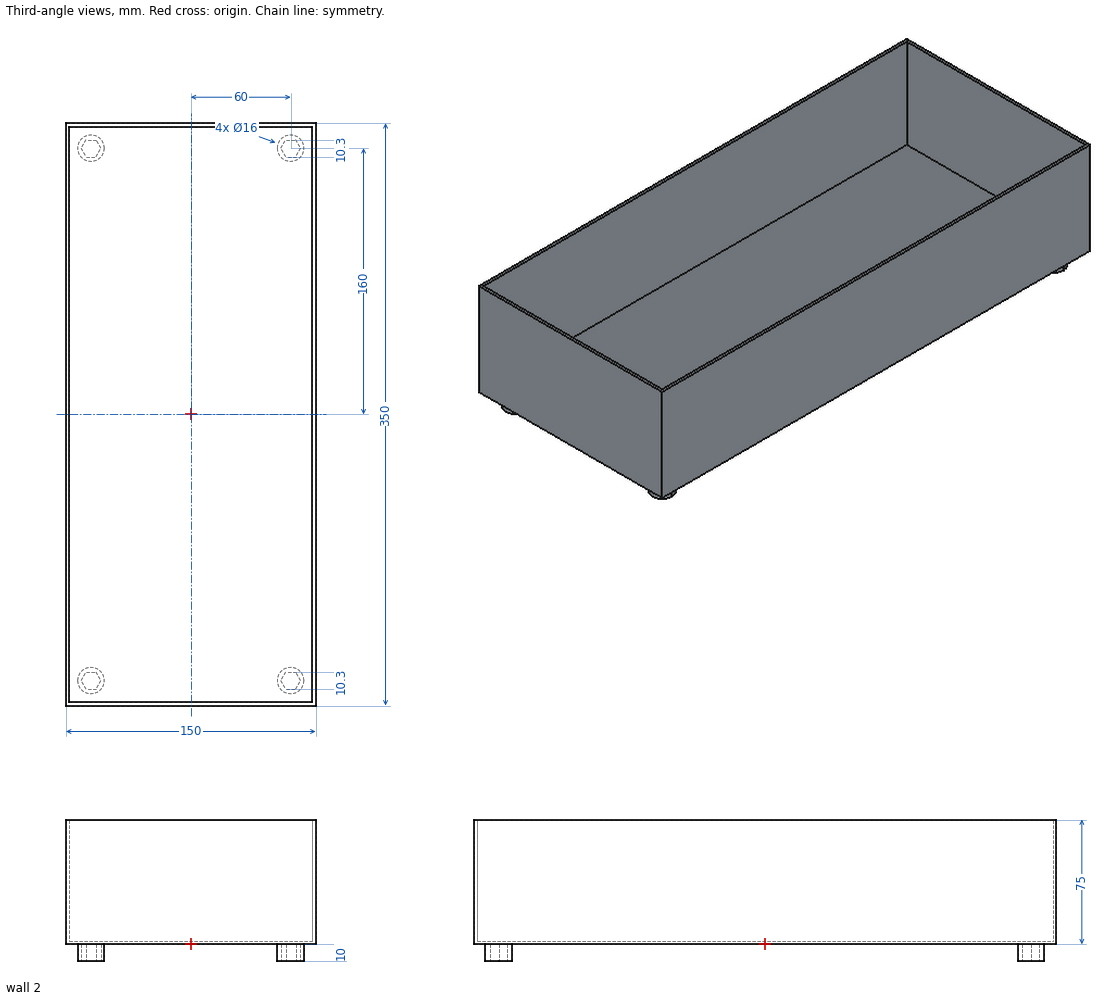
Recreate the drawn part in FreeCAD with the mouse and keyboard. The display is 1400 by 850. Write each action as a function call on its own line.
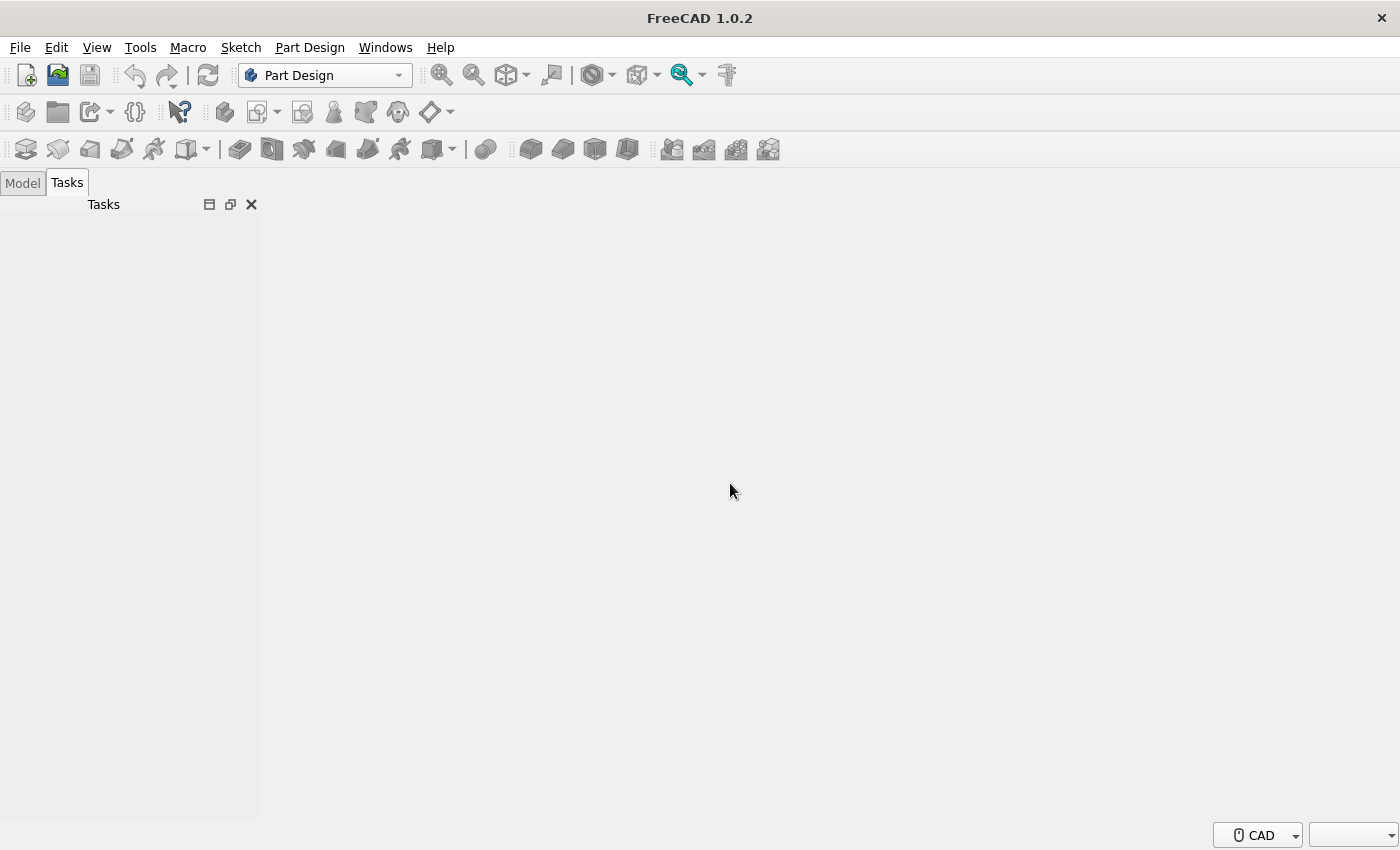
click(26, 76)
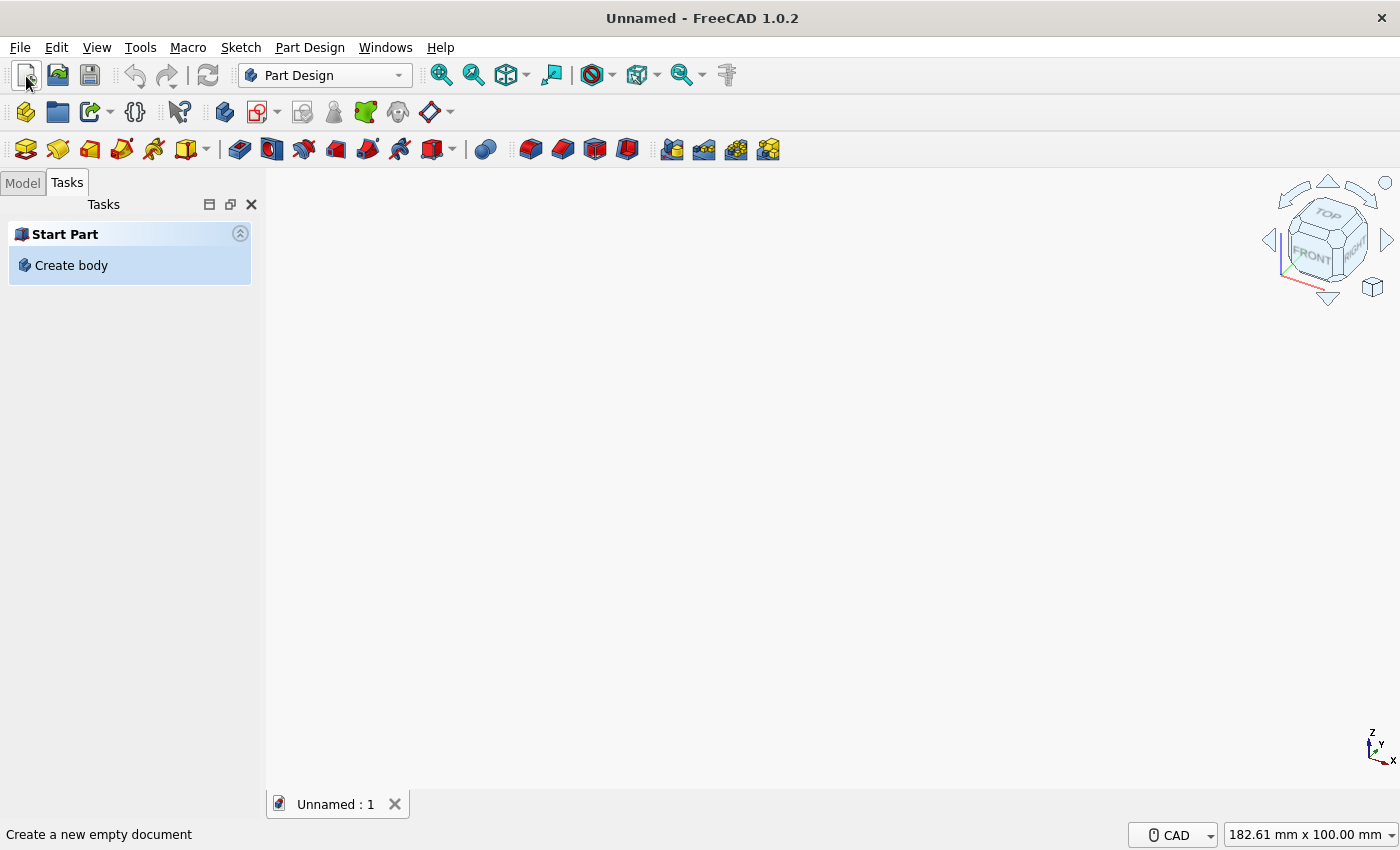
click(258, 112)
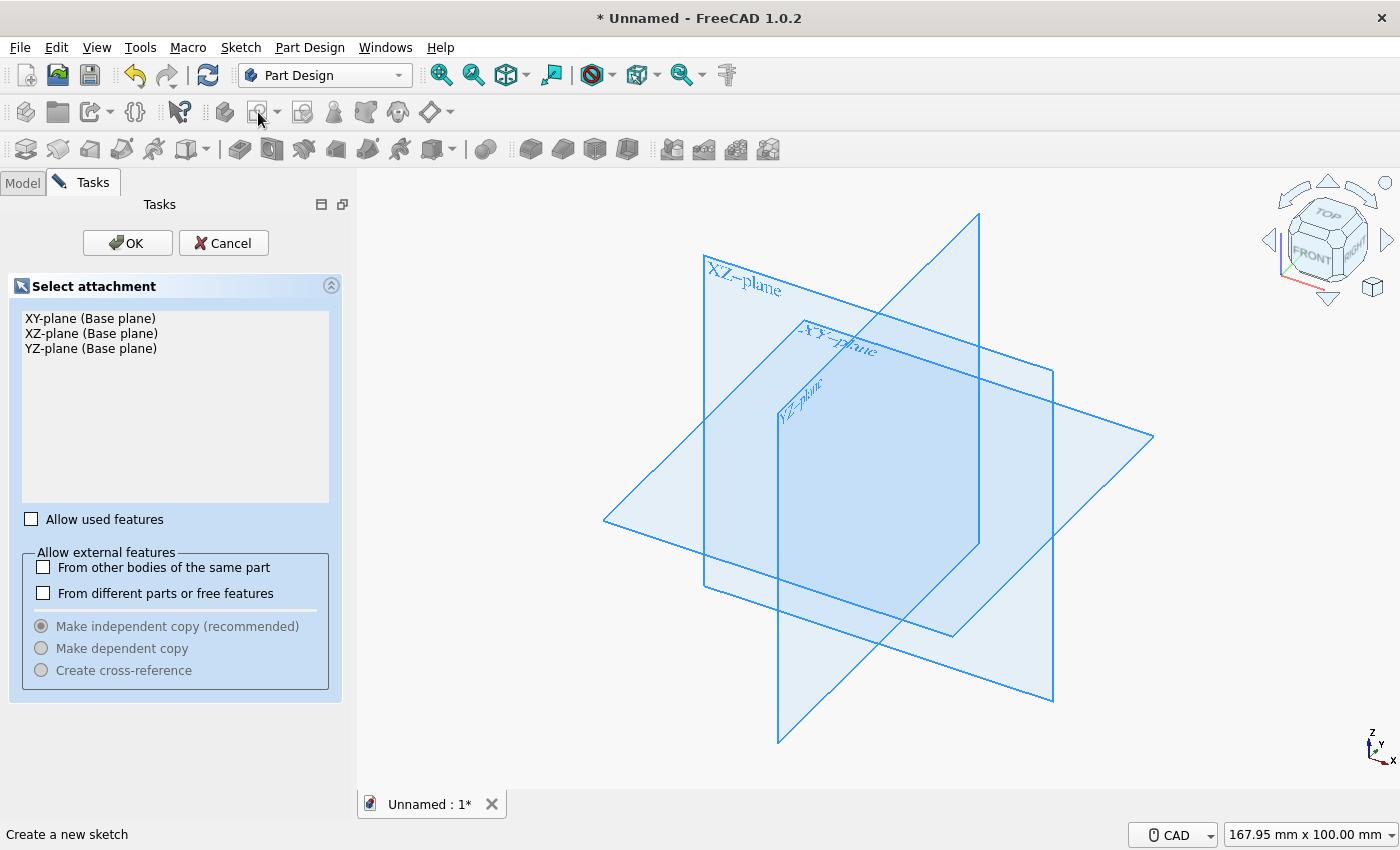
click(82, 318)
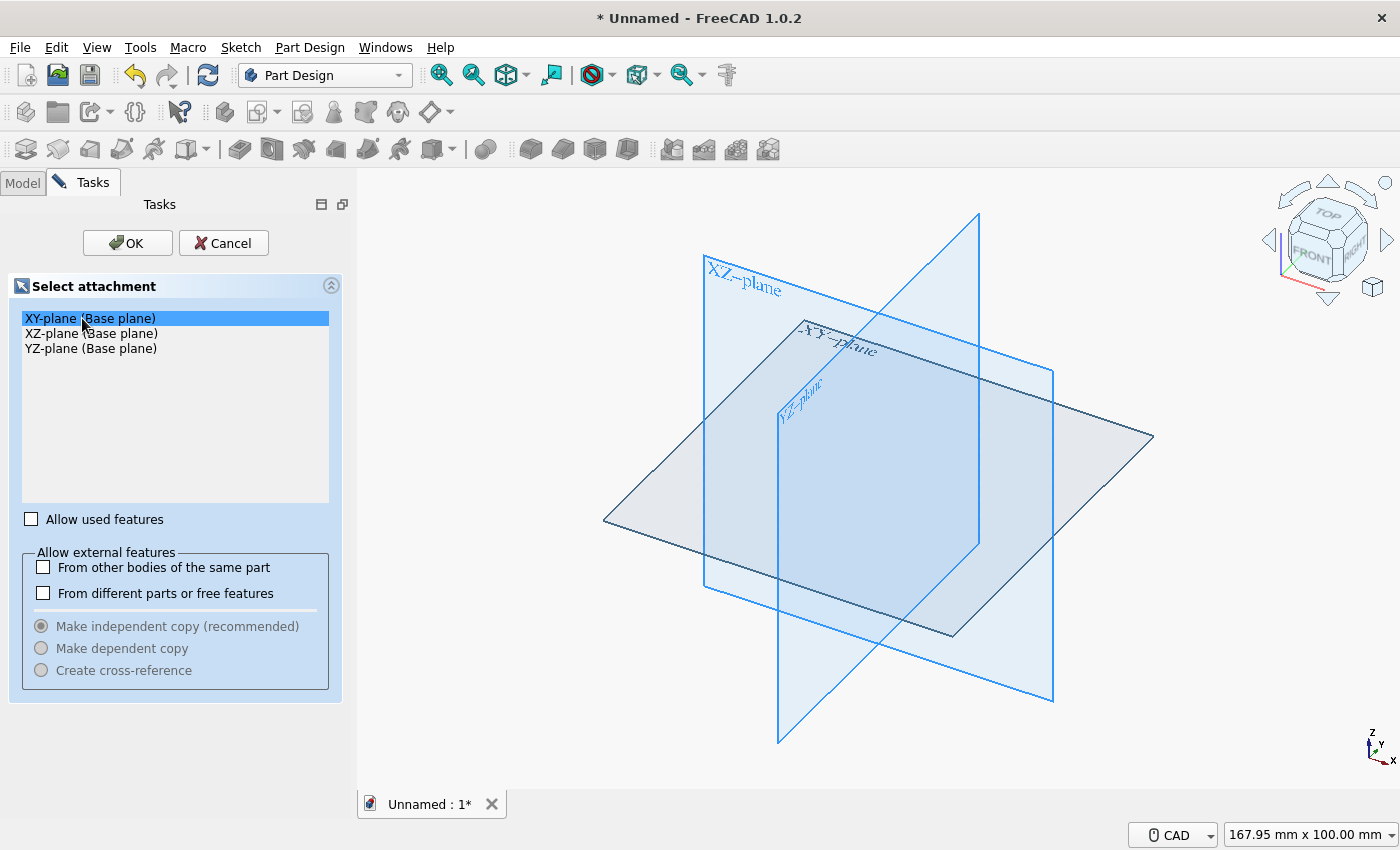
click(128, 243)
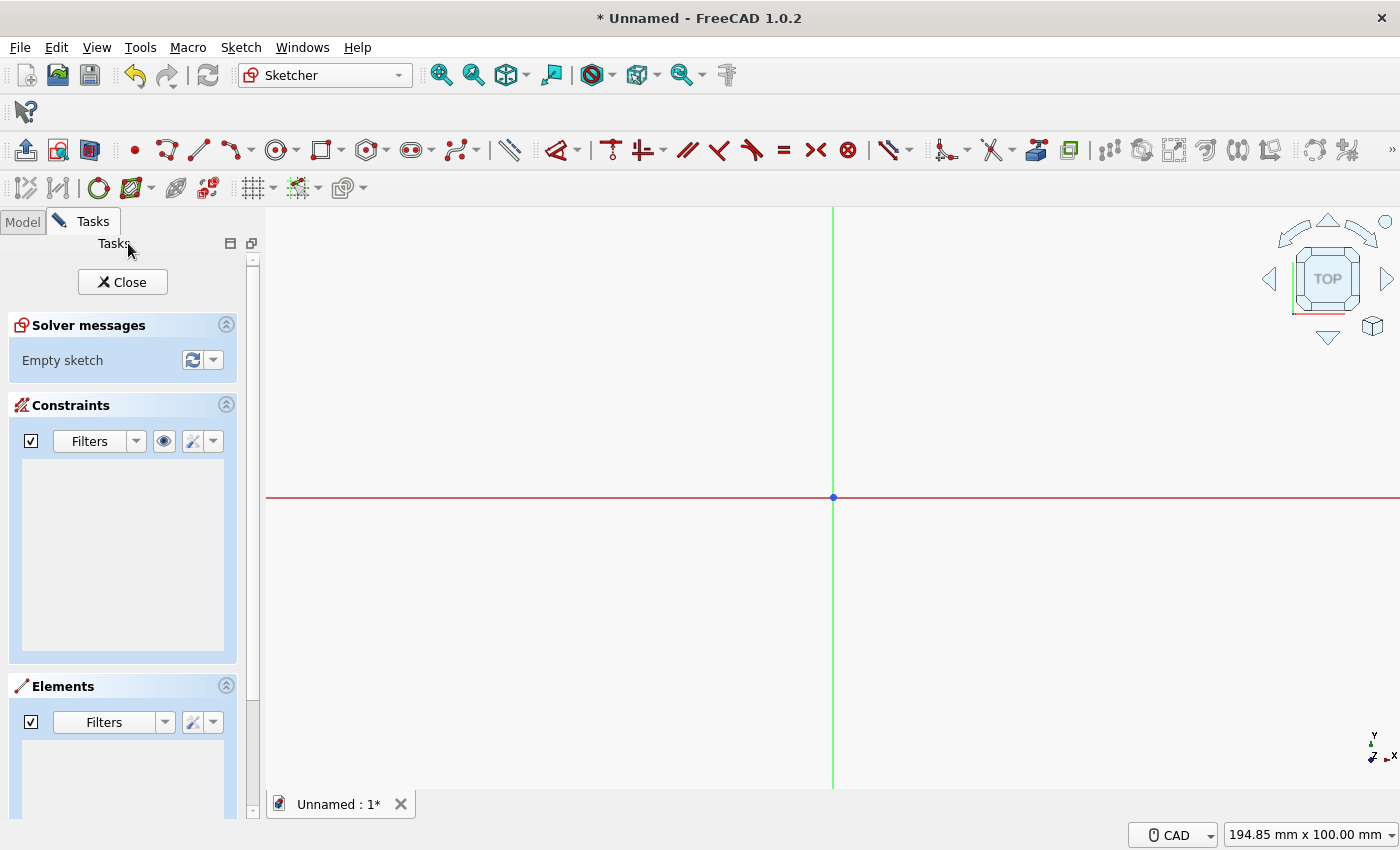
scroll(751, 498, down, 9)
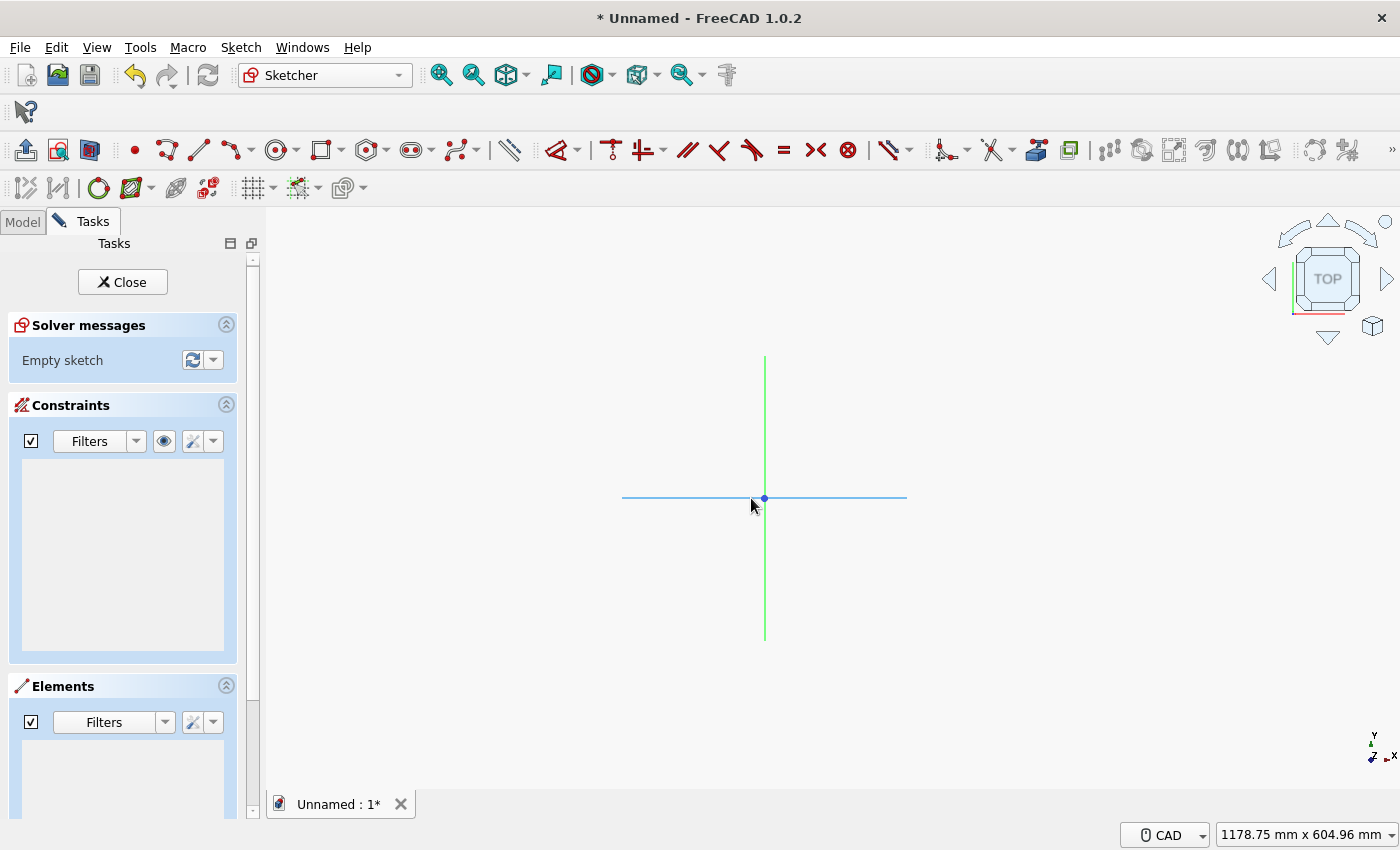
key(g)
key(v)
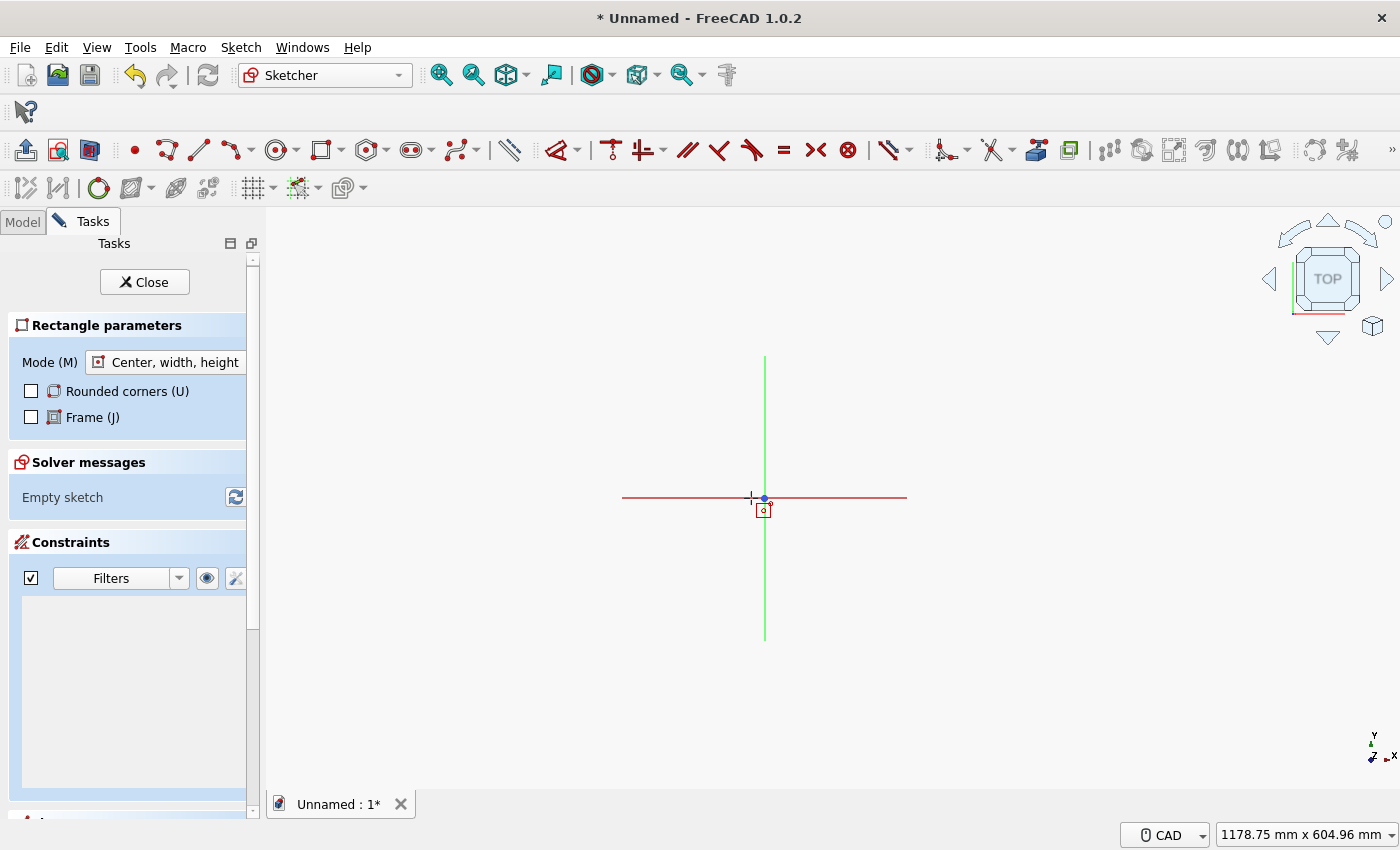
click(765, 498)
move(837, 330)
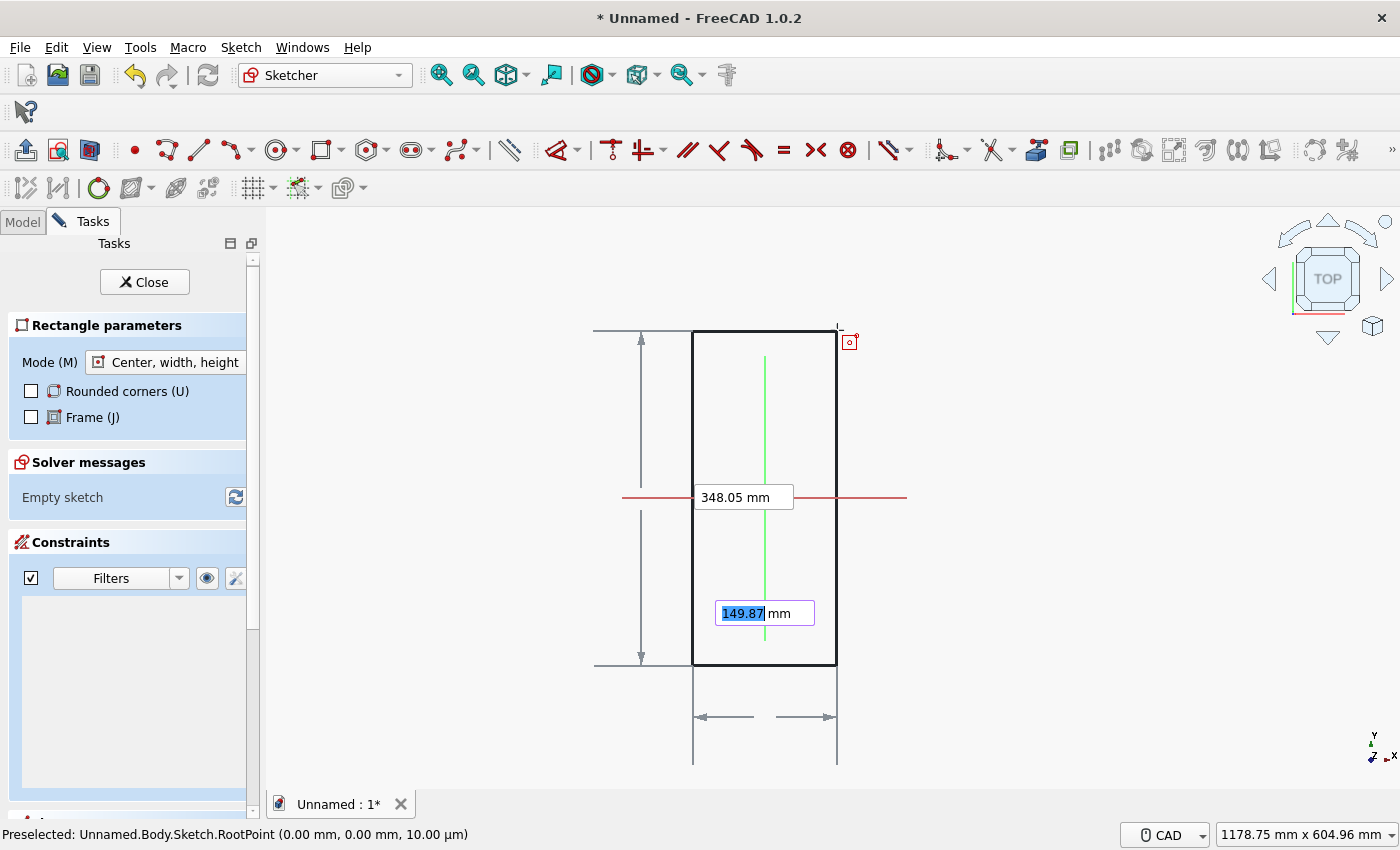
text(150)
key(Tab)
text(350)
key(Return)
key(Escape)